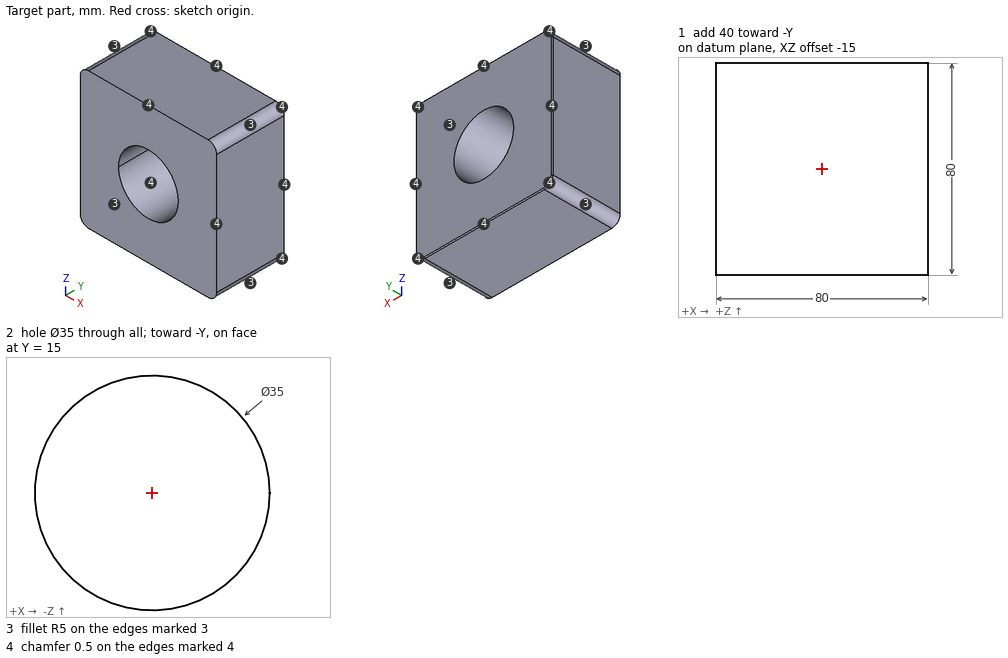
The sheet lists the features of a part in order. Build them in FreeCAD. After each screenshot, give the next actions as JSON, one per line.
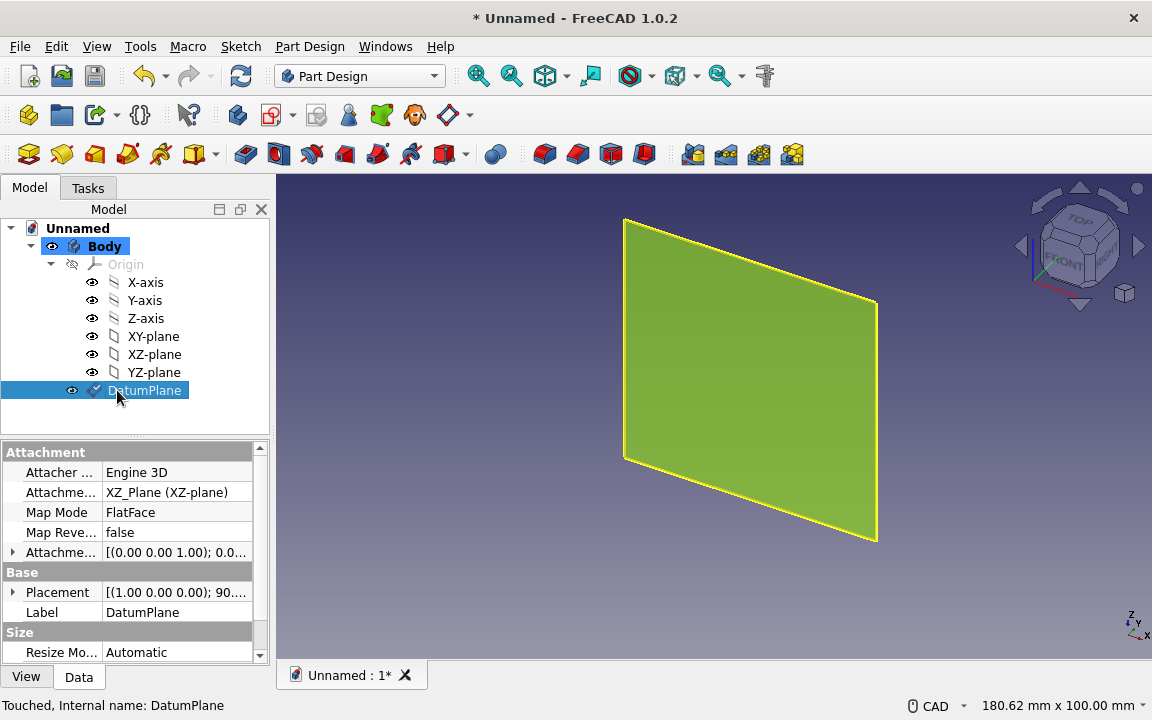
{"action": "left_click", "coordinate": [270, 116]}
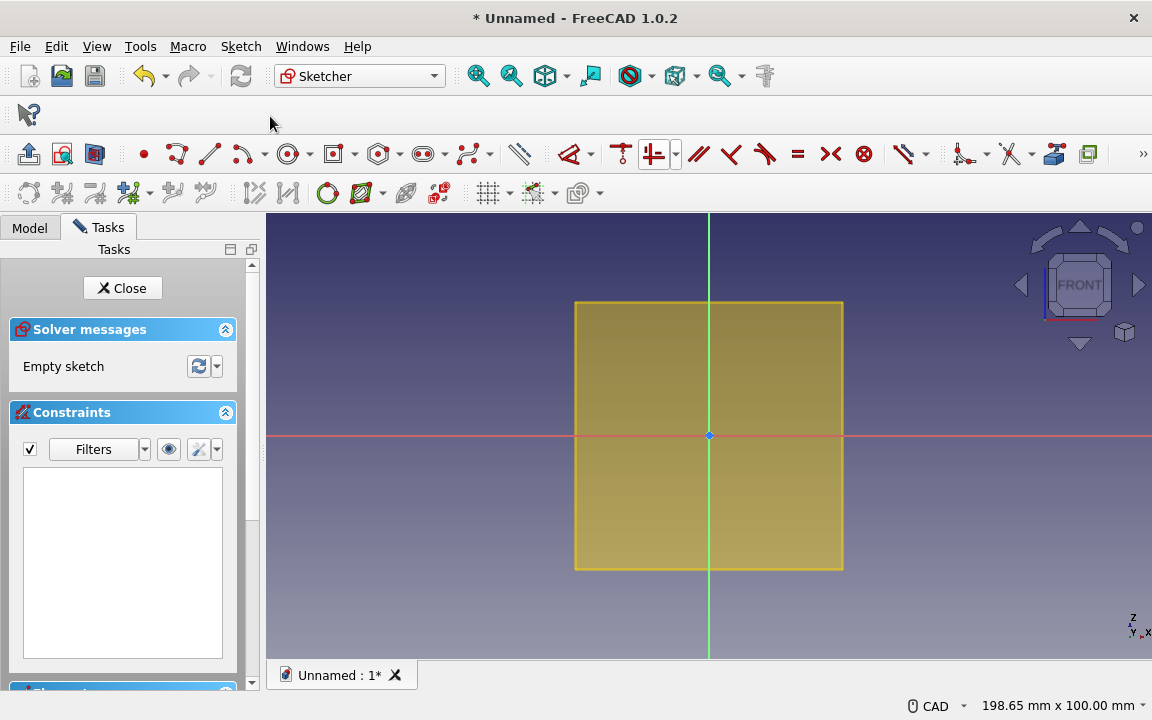
{"action": "scroll", "coordinate": [331, 436], "scroll_direction": "down", "scroll_amount": 1}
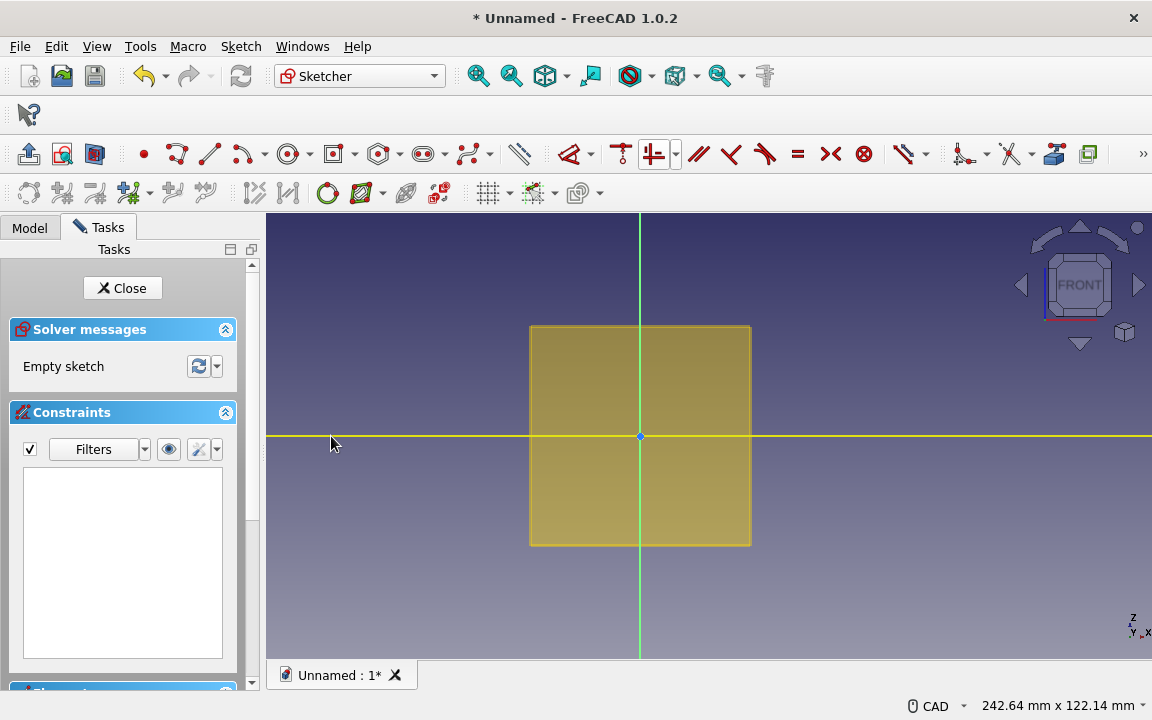
{"action": "left_click", "coordinate": [332, 154]}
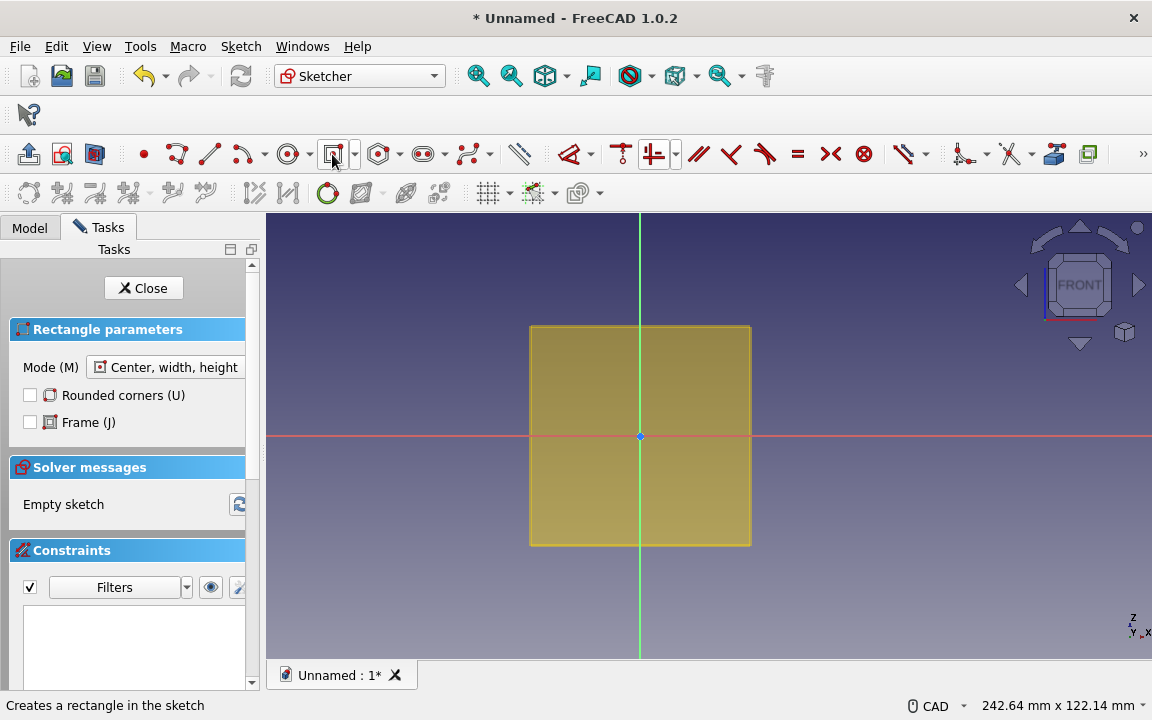
{"action": "left_click", "coordinate": [640, 436]}
{"action": "left_click", "coordinate": [787, 290]}
{"action": "key", "text": "Escape"}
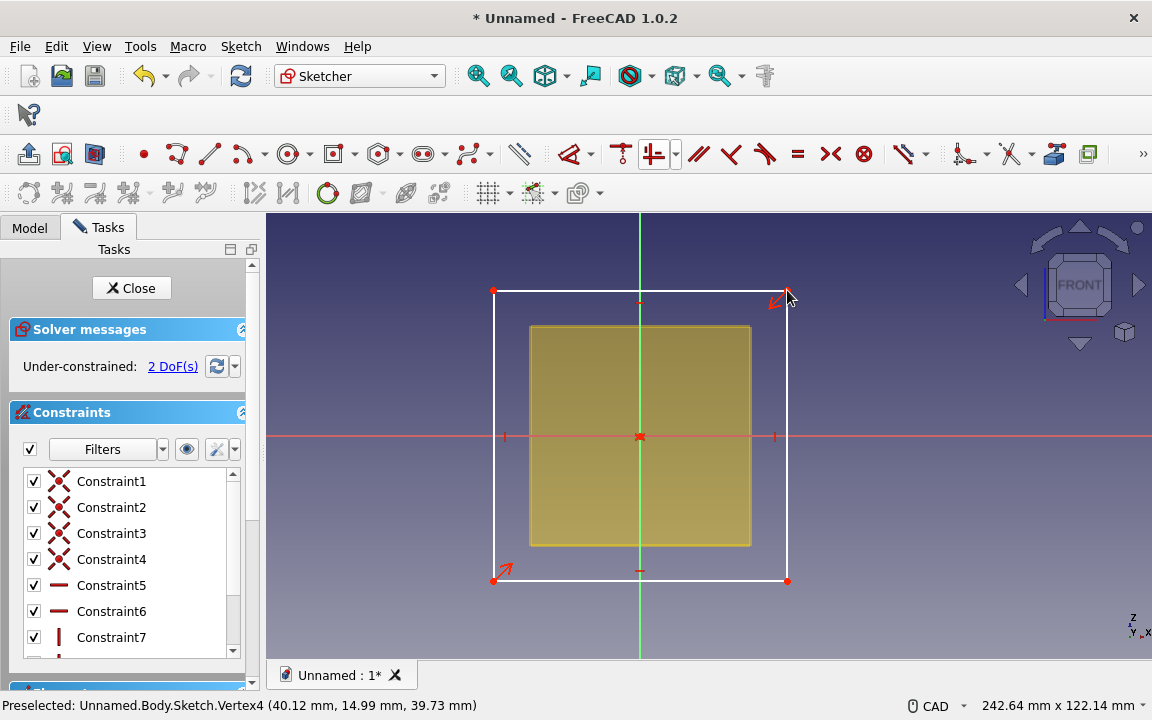
{"action": "left_click", "coordinate": [568, 154]}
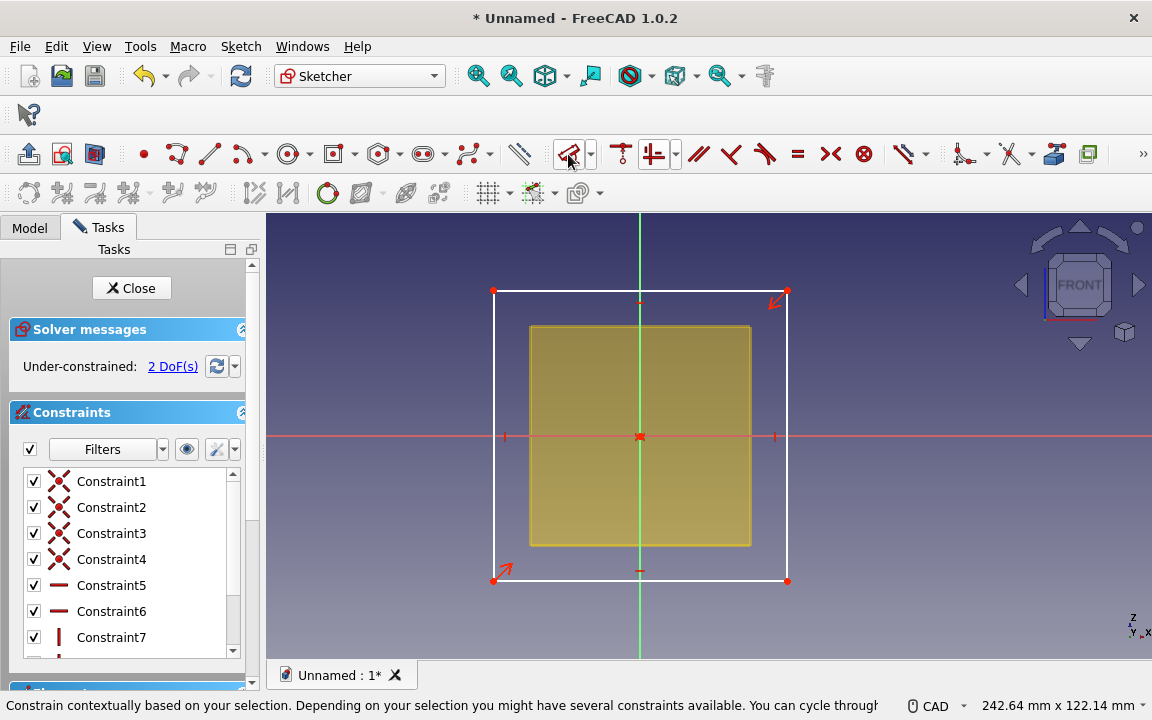
{"action": "left_click", "coordinate": [582, 581]}
{"action": "left_click", "coordinate": [573, 615]}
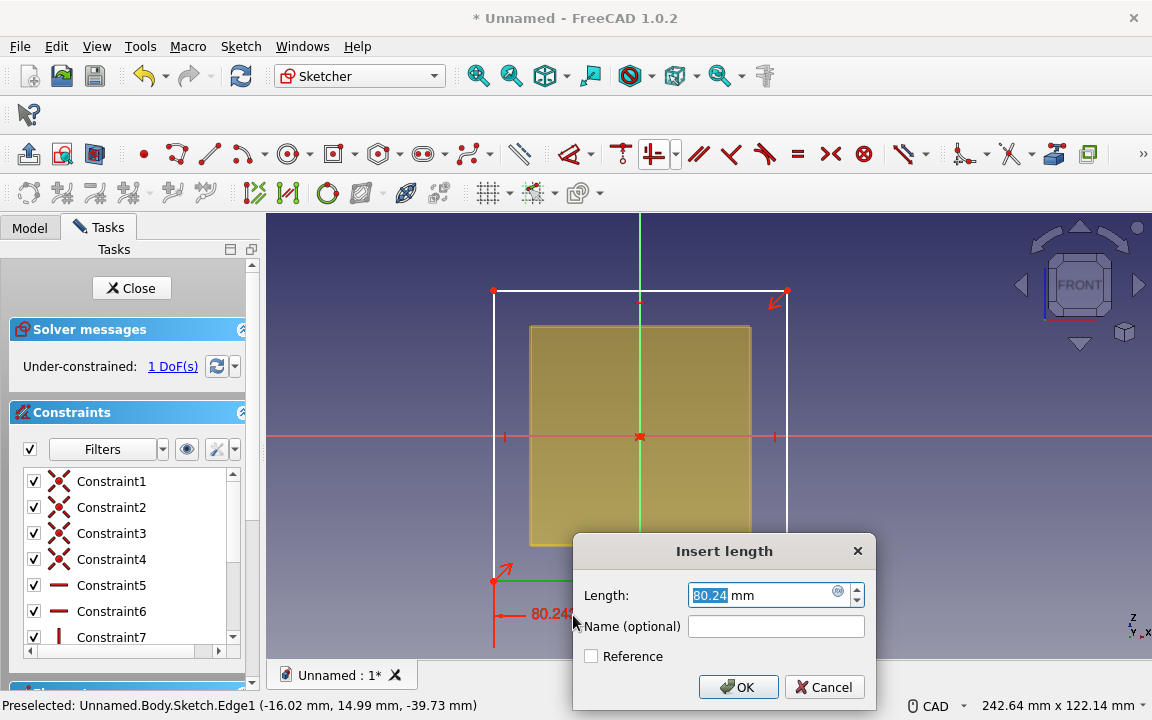
{"action": "type", "text": "80"}
{"action": "key", "text": "Return"}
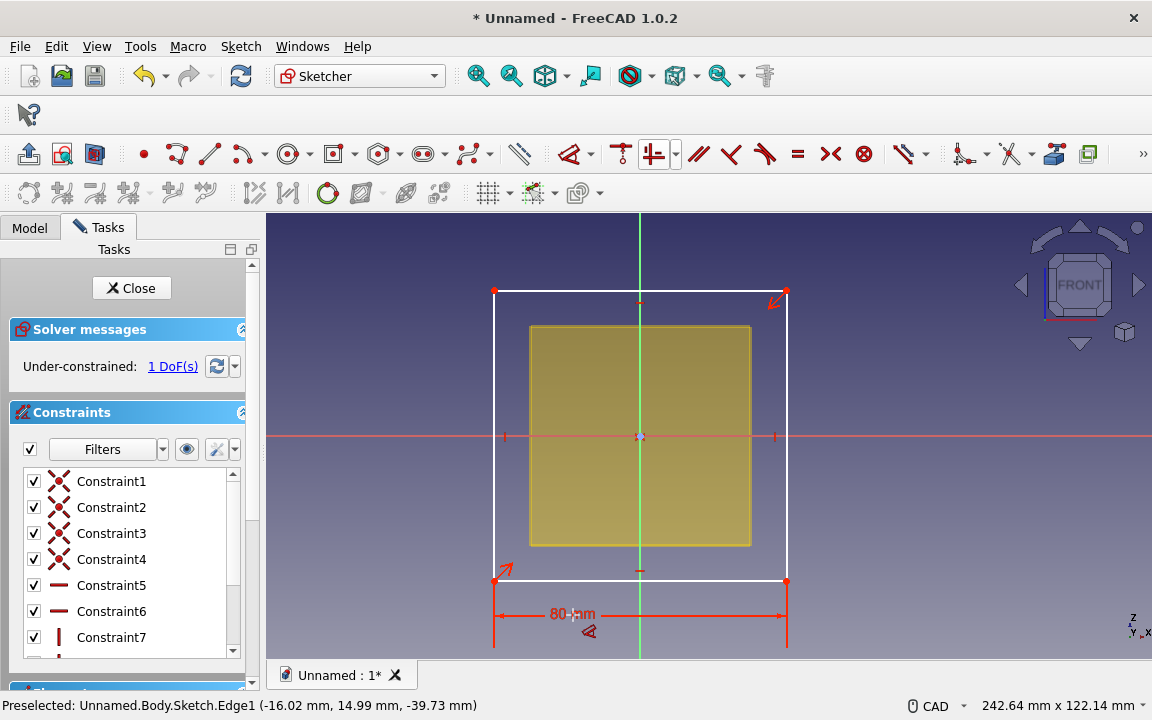
{"action": "left_click", "coordinate": [787, 494]}
{"action": "left_click", "coordinate": [821, 369]}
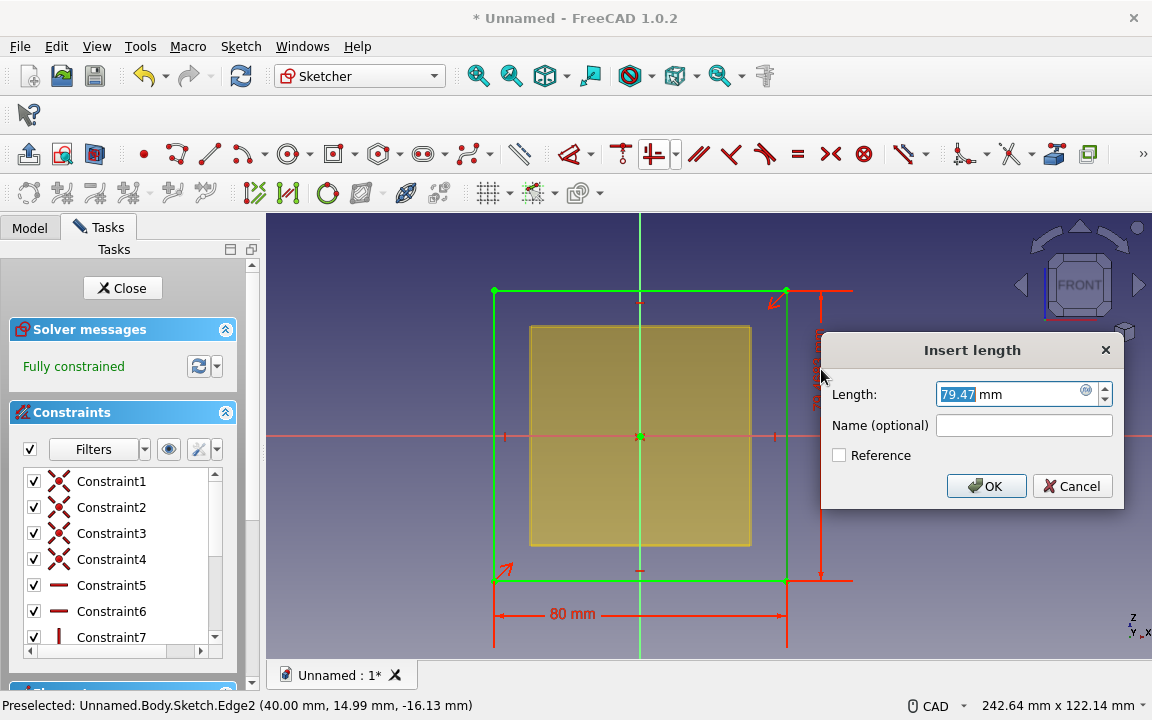
{"action": "type", "text": "80"}
{"action": "key", "text": "Return"}
{"action": "key", "text": "Escape"}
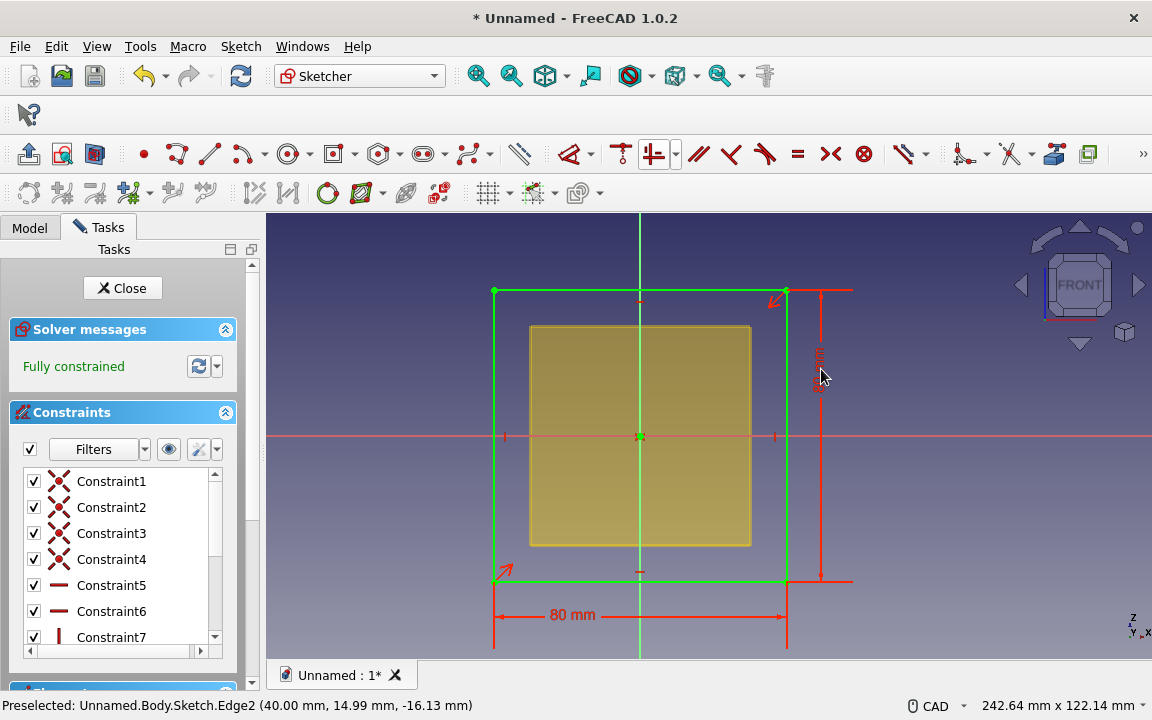
{"action": "left_click", "coordinate": [123, 288]}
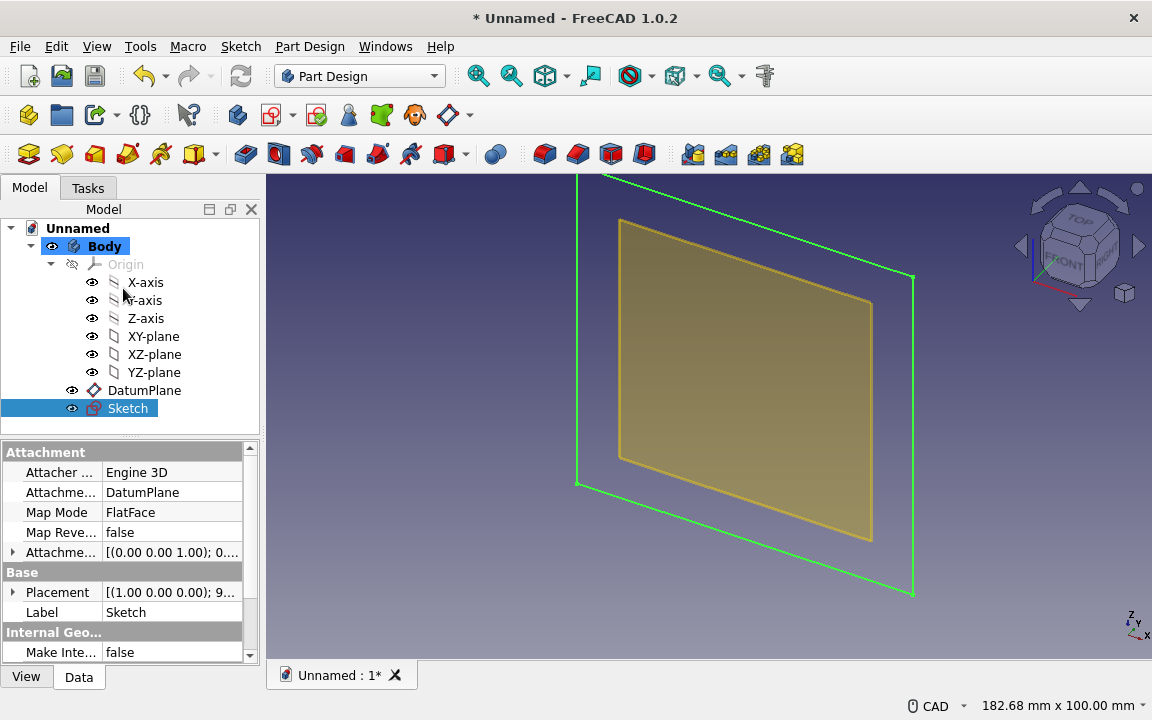
{"action": "left_click", "coordinate": [29, 154]}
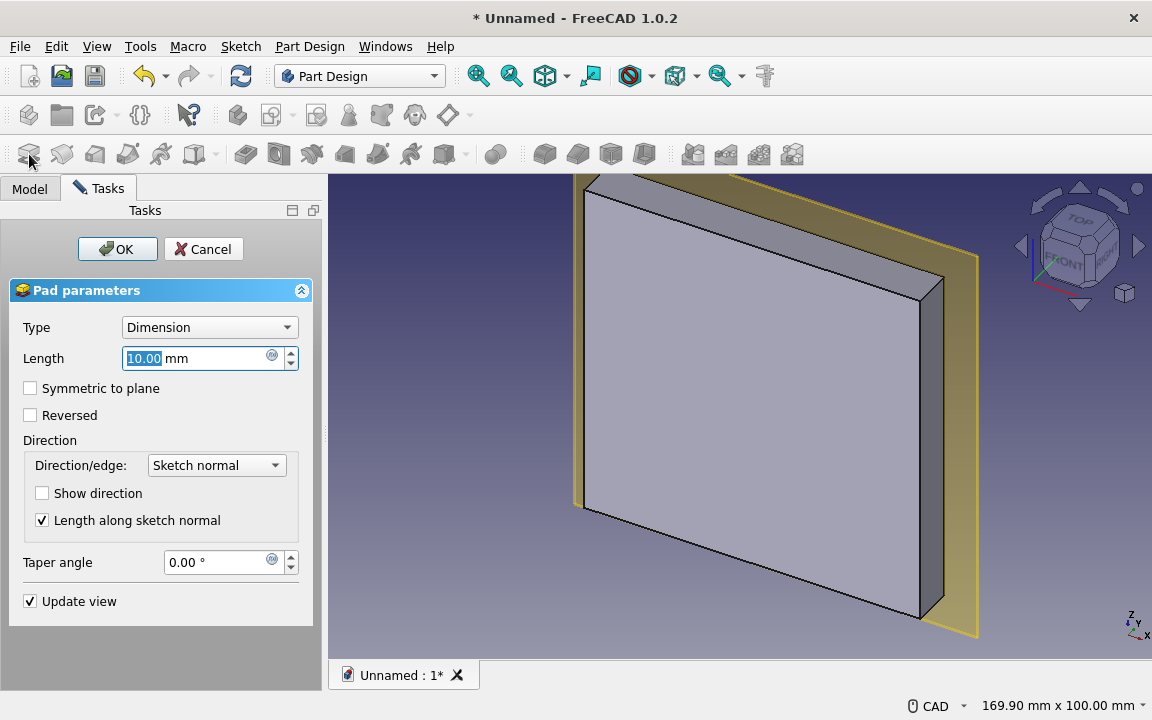
{"action": "type", "text": "40"}
{"action": "key", "text": "Tab"}